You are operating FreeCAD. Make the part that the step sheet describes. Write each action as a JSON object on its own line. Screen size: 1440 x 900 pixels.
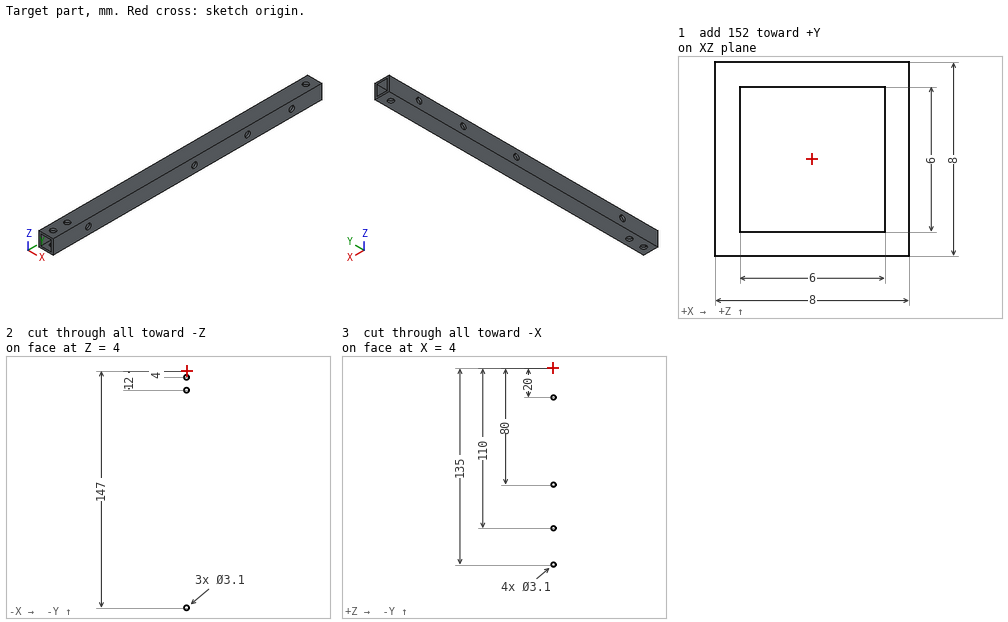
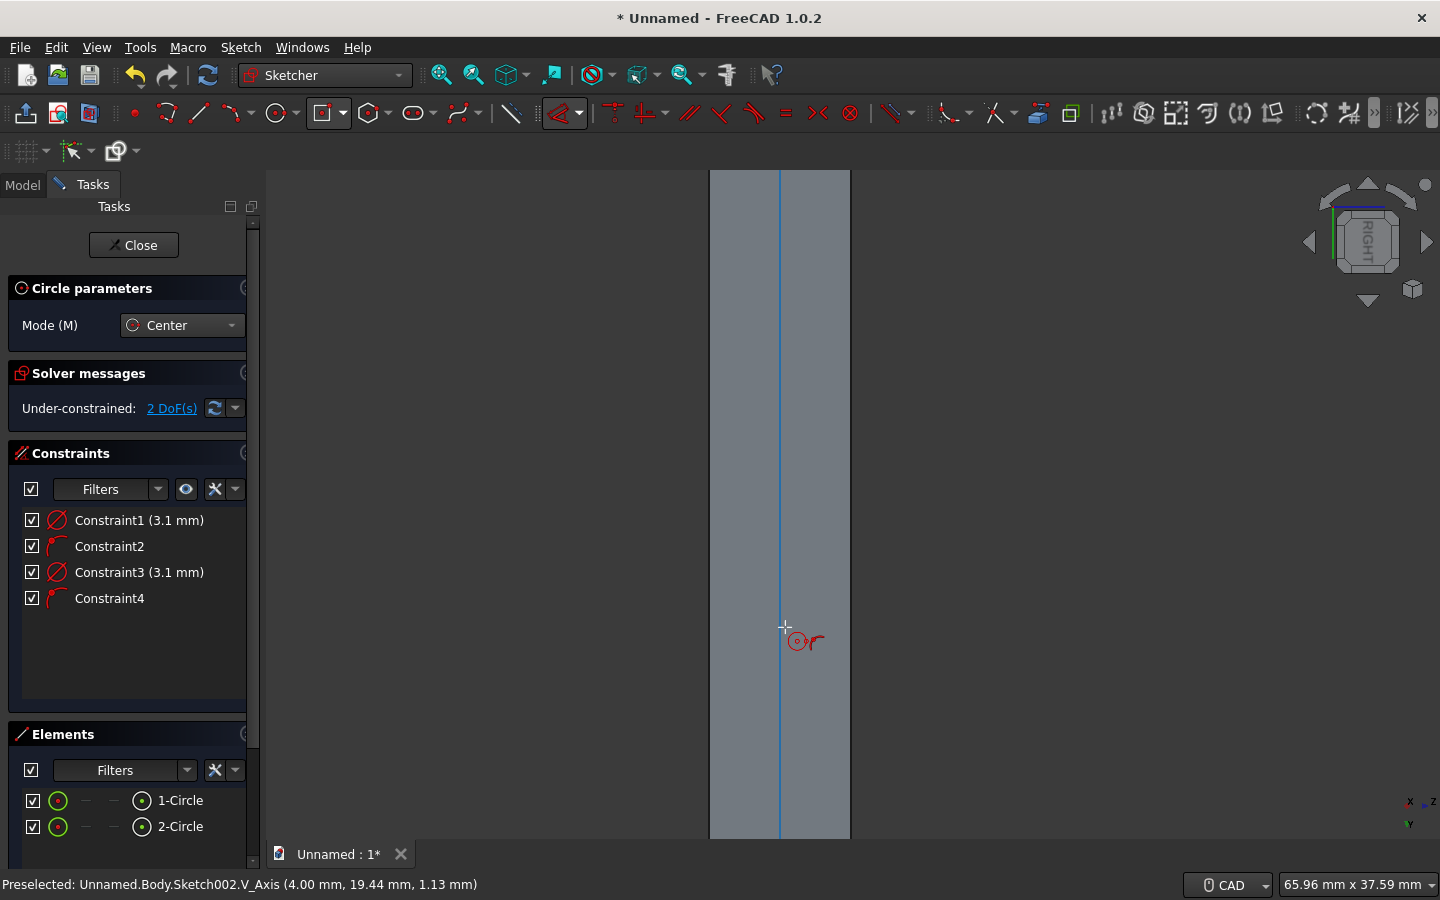
{"action": "scroll", "coordinate": [785, 628], "scroll_direction": "down", "scroll_amount": 9}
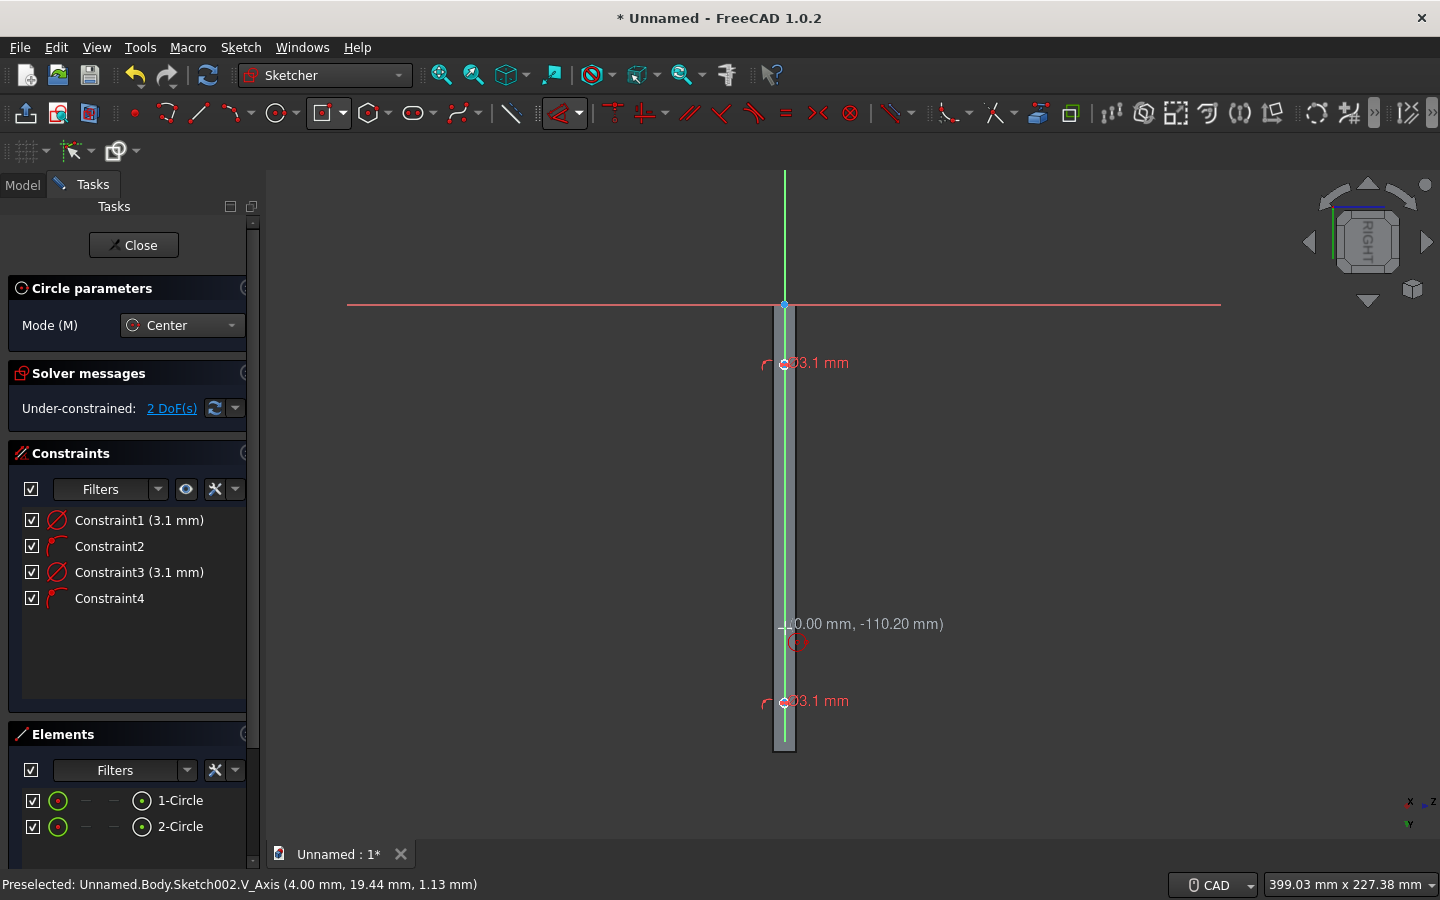
{"action": "left_click", "coordinate": [785, 628]}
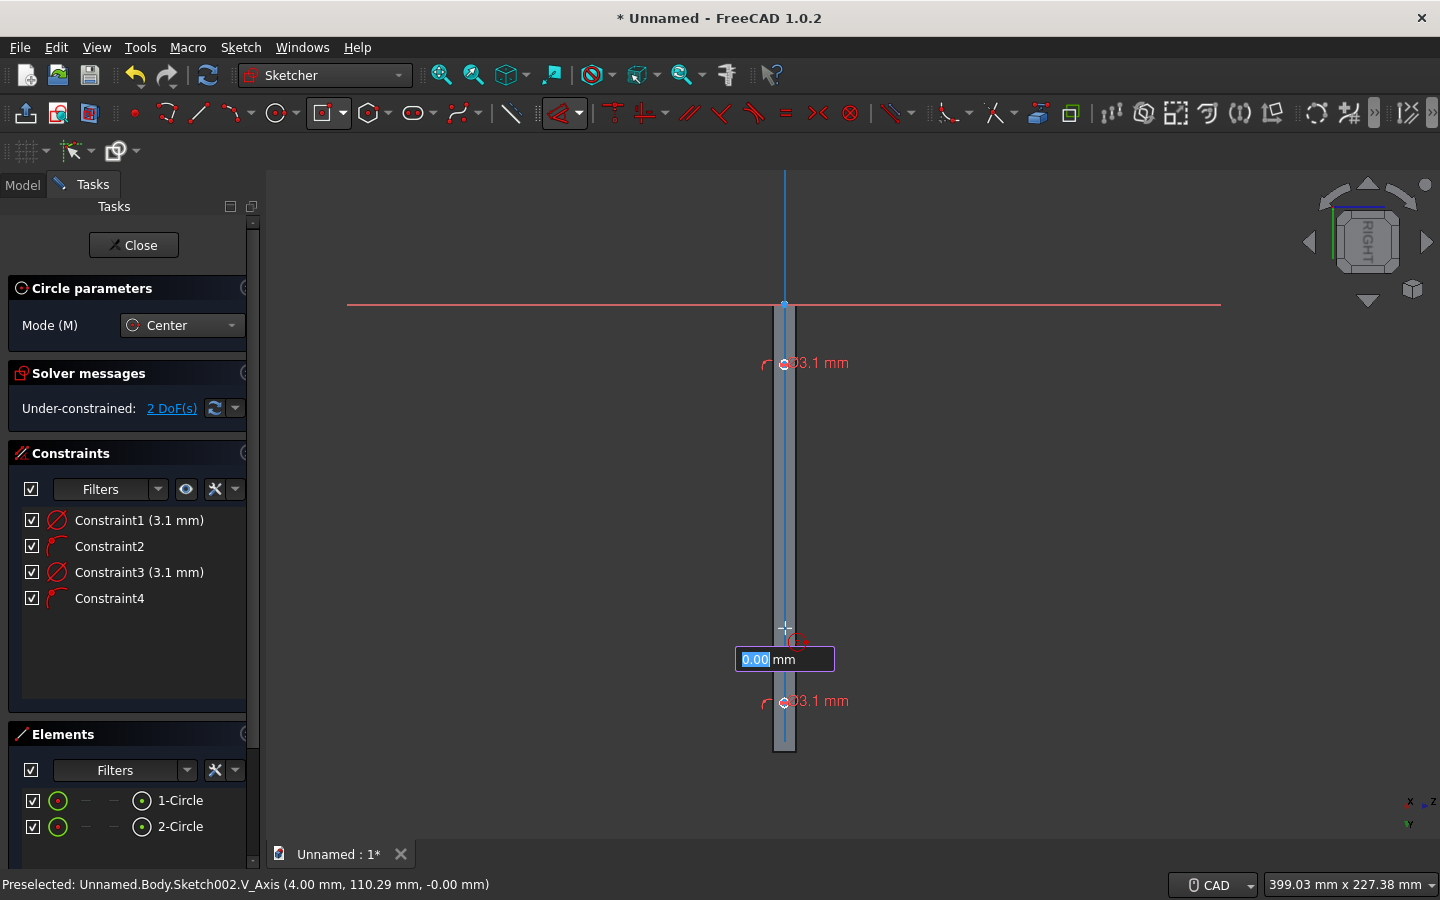
{"action": "scroll", "coordinate": [789, 627], "scroll_direction": "up", "scroll_amount": 7}
{"action": "mouse_move", "coordinate": [787, 623]}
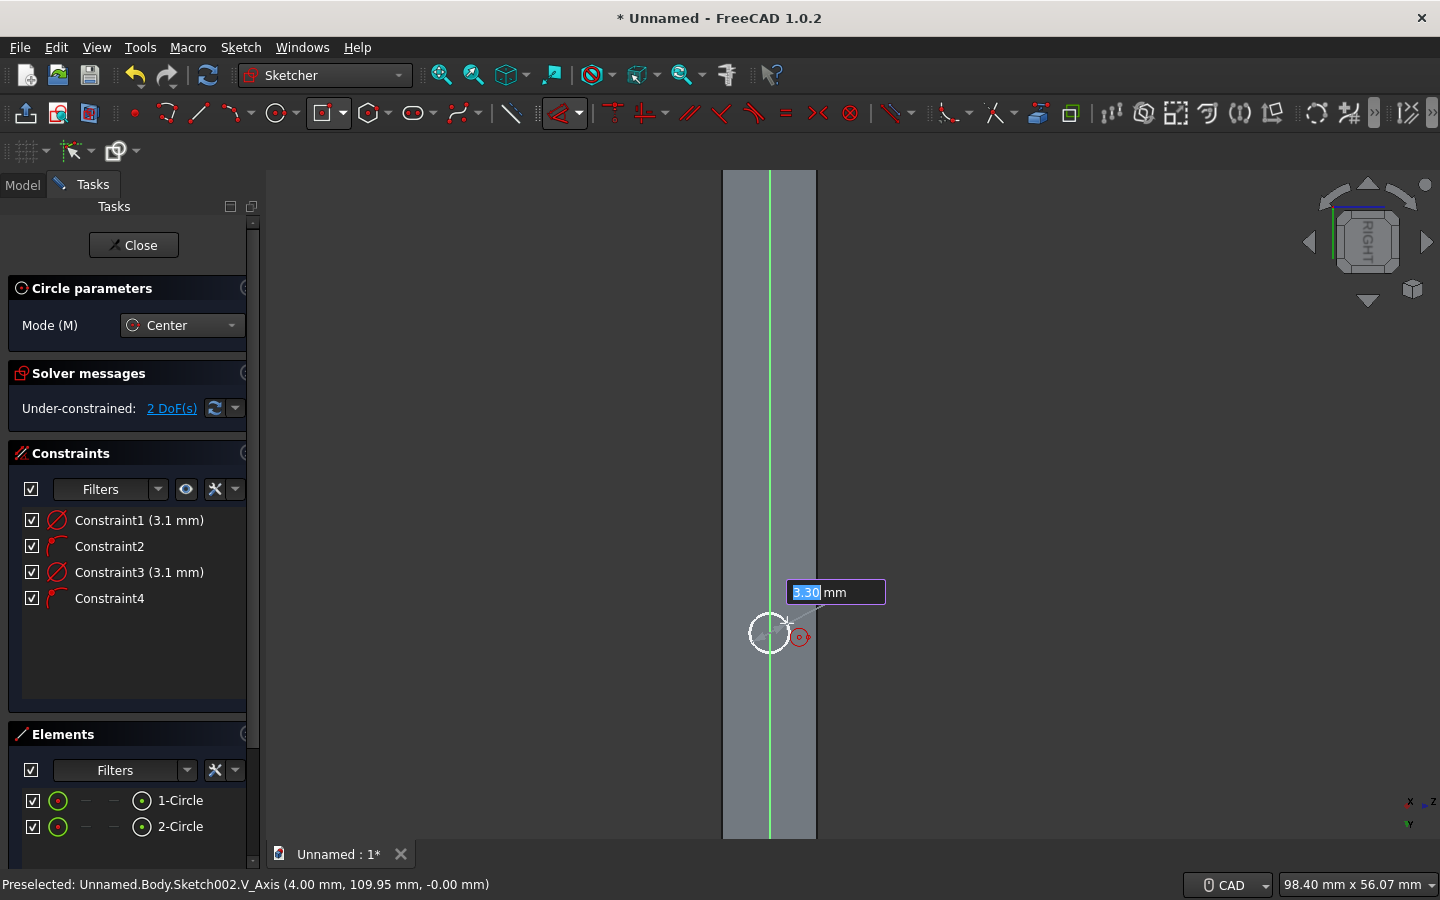
{"action": "type", "text": "3.1"}
{"action": "key", "text": "Return"}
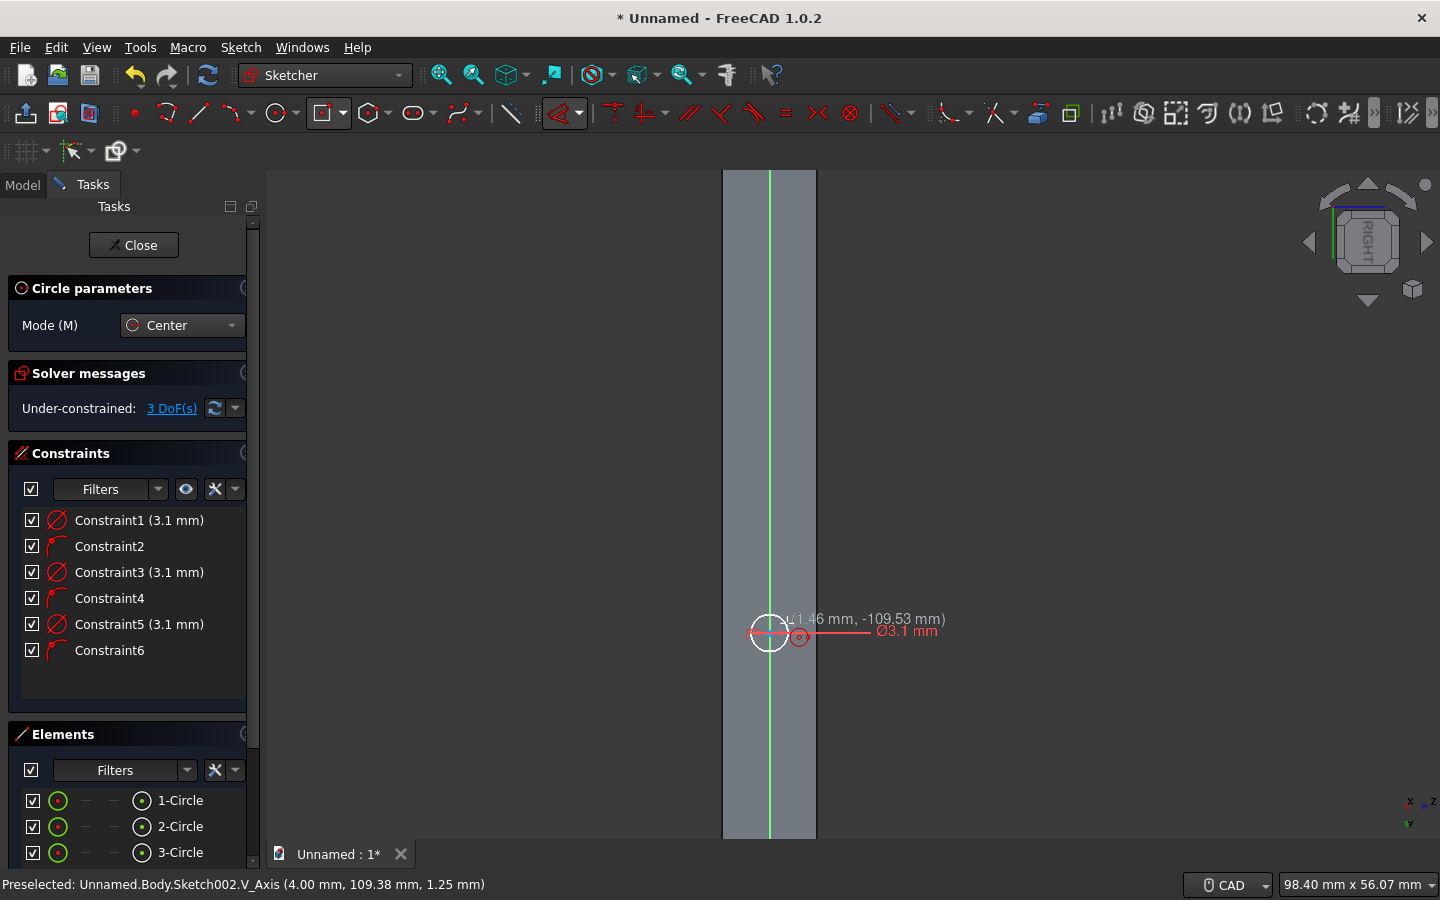
{"action": "scroll", "coordinate": [770, 272], "scroll_direction": "up", "scroll_amount": 2}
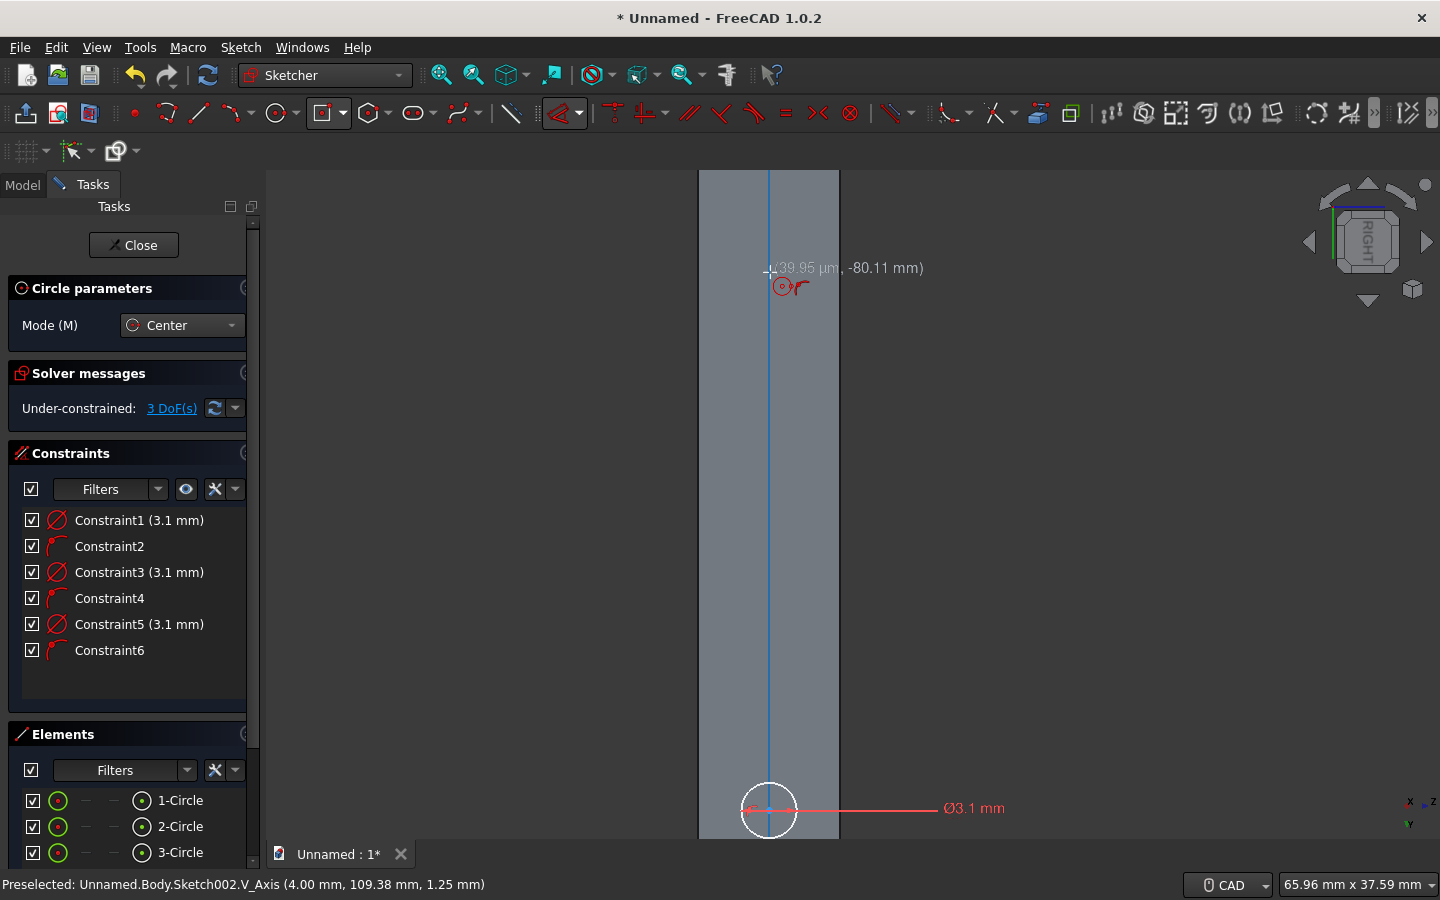
{"action": "scroll", "coordinate": [788, 592], "scroll_direction": "down", "scroll_amount": 9}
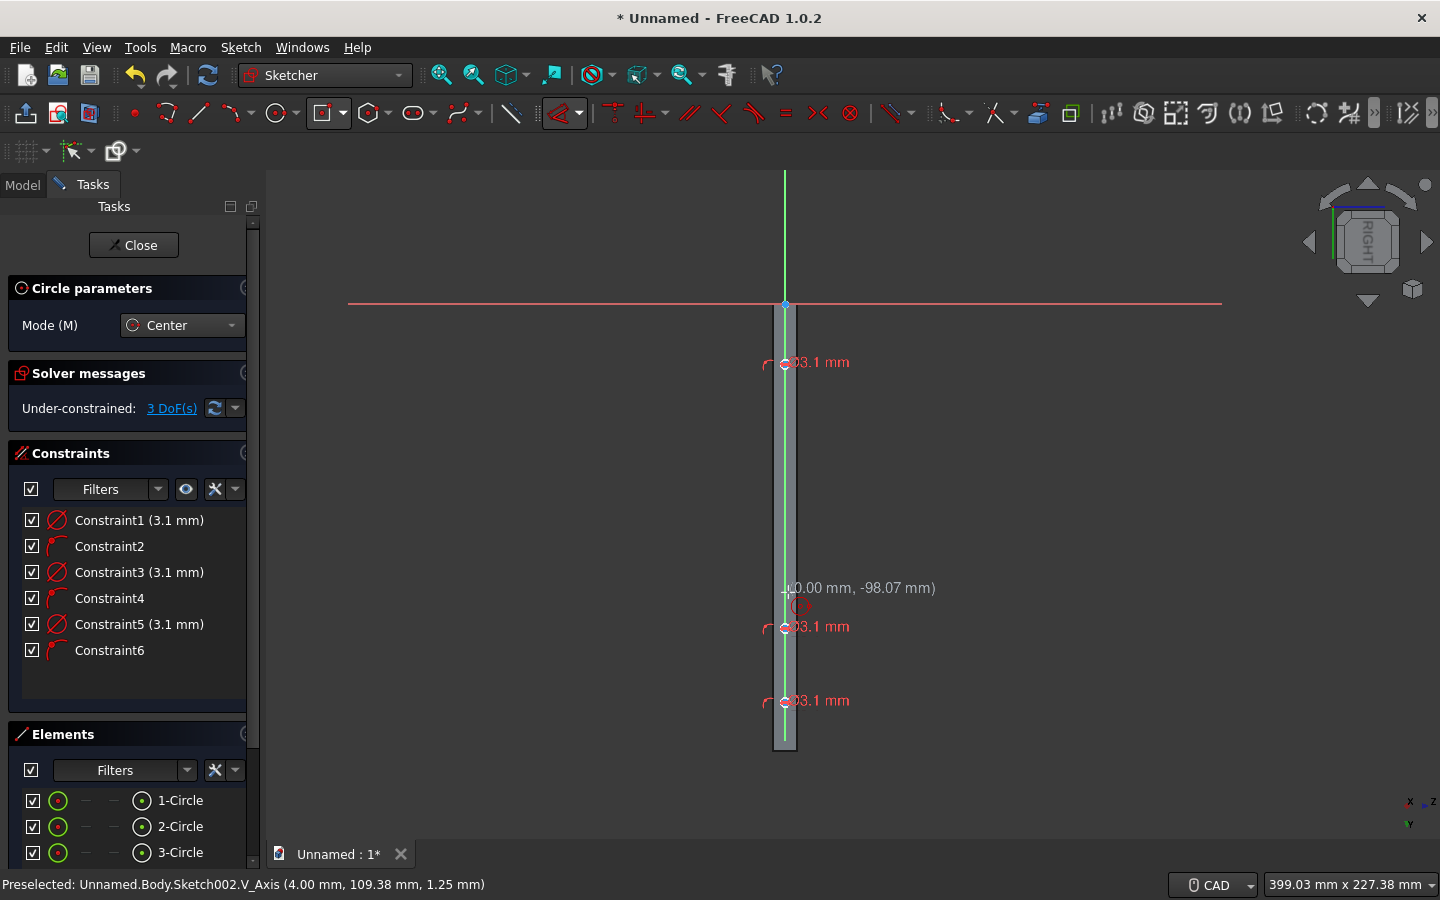
{"action": "left_click", "coordinate": [785, 540]}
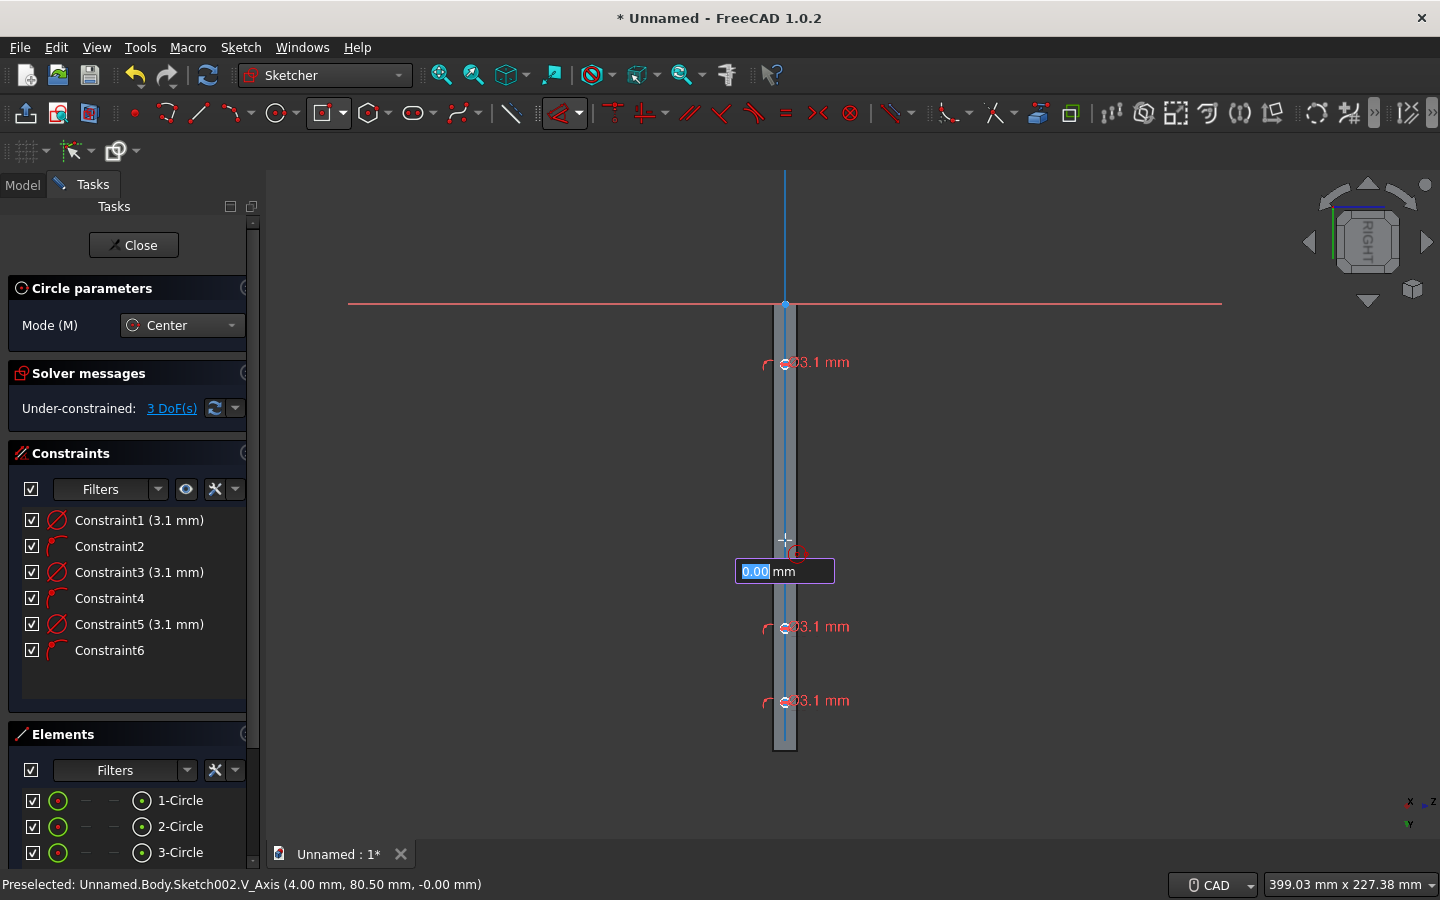
{"action": "scroll", "coordinate": [790, 538], "scroll_direction": "up", "scroll_amount": 7}
{"action": "mouse_move", "coordinate": [787, 536]}